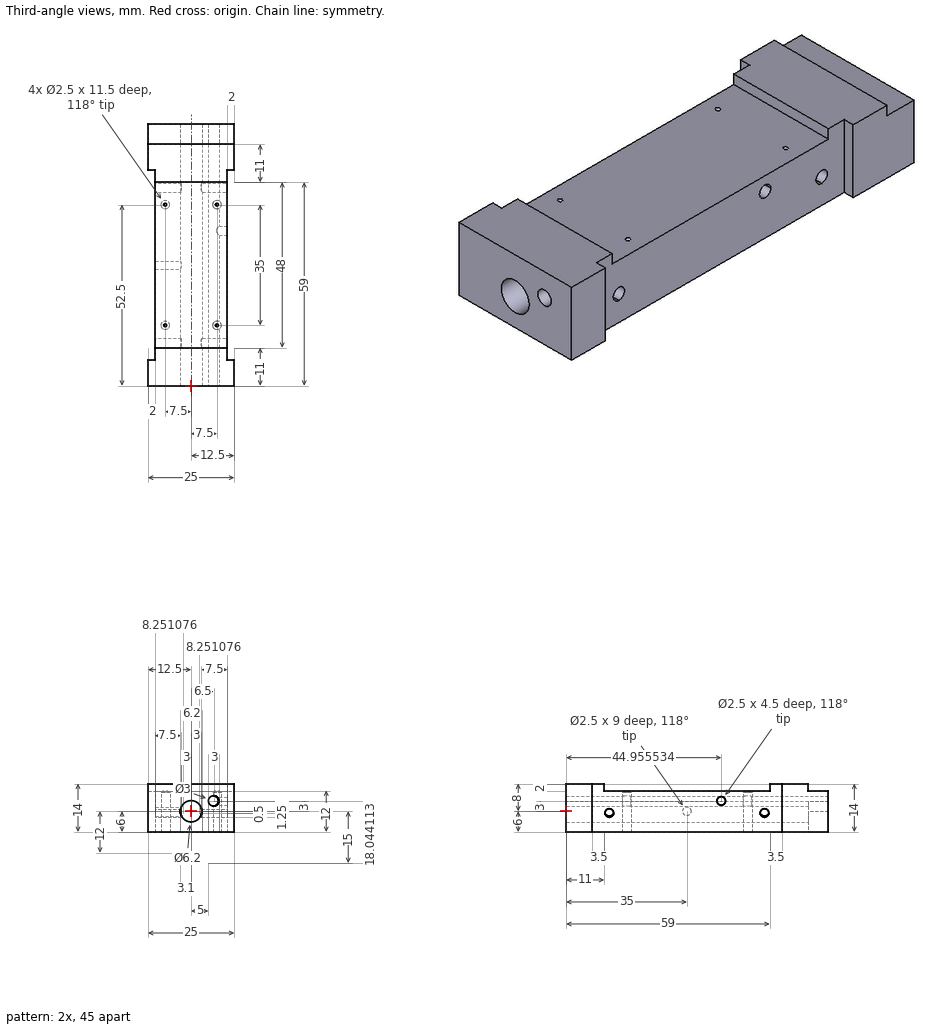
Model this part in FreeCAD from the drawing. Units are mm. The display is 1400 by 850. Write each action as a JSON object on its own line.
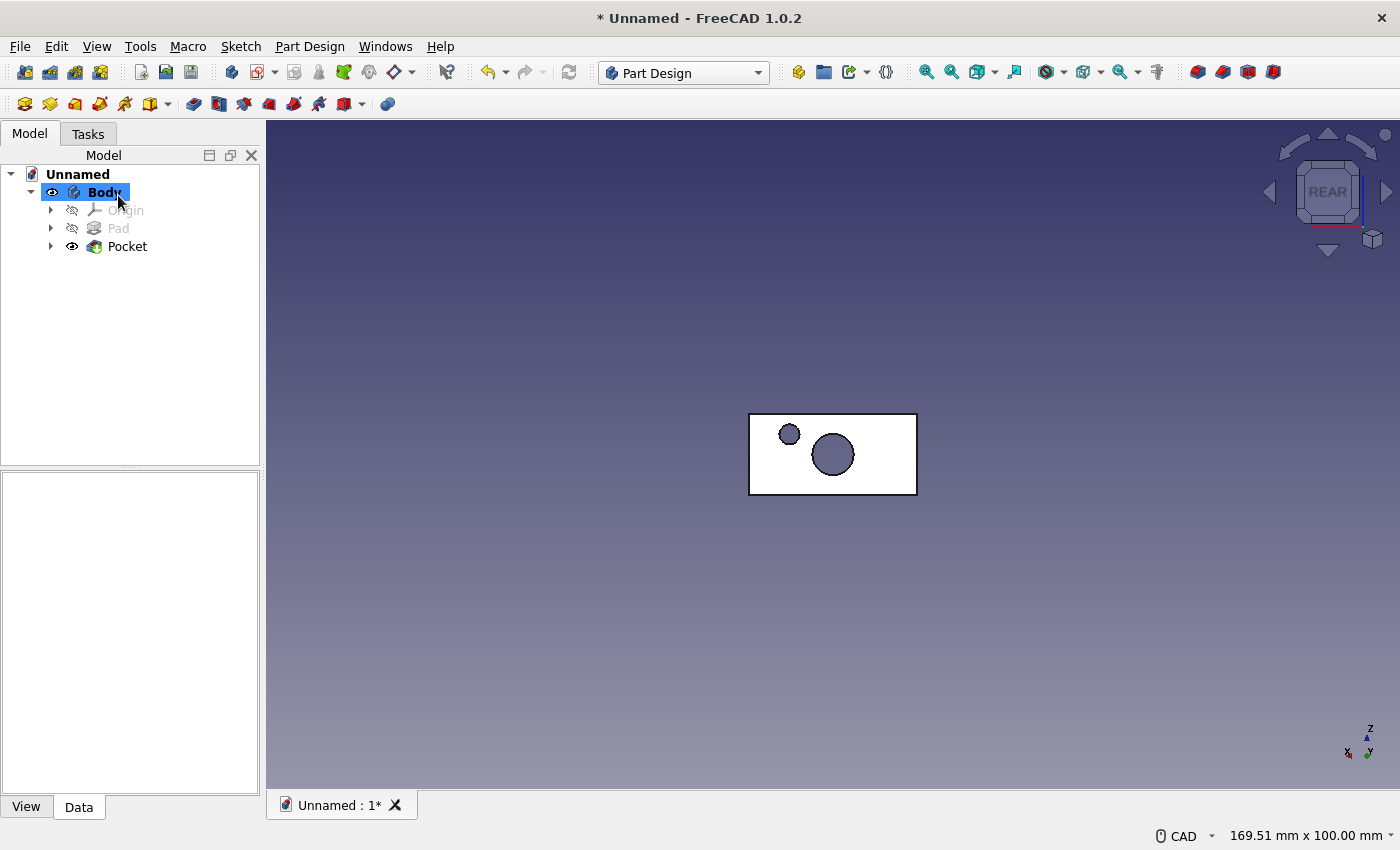
{"action": "left_click", "coordinate": [927, 72]}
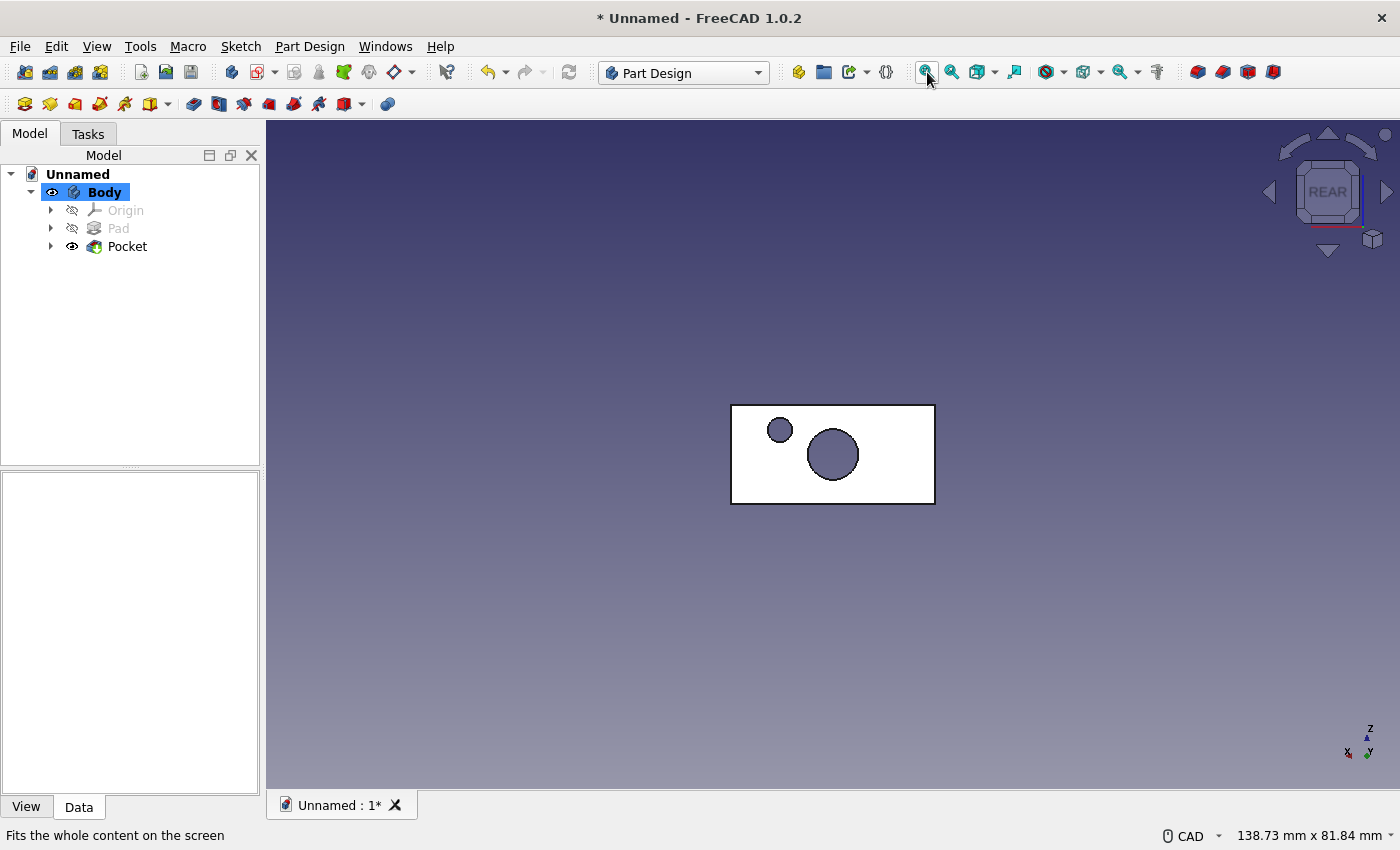
{"action": "left_click", "coordinate": [891, 439]}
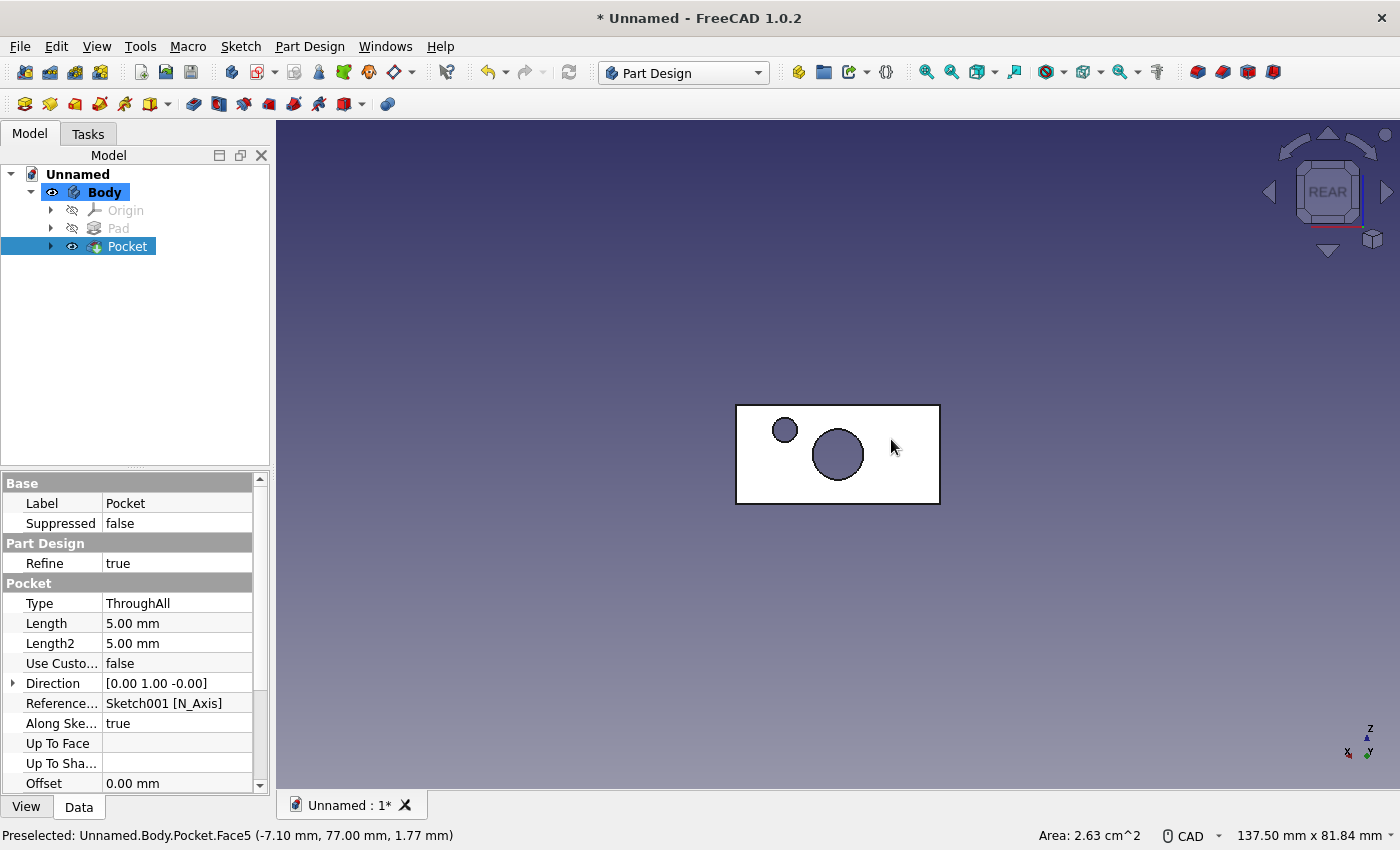
{"action": "left_click", "coordinate": [256, 72]}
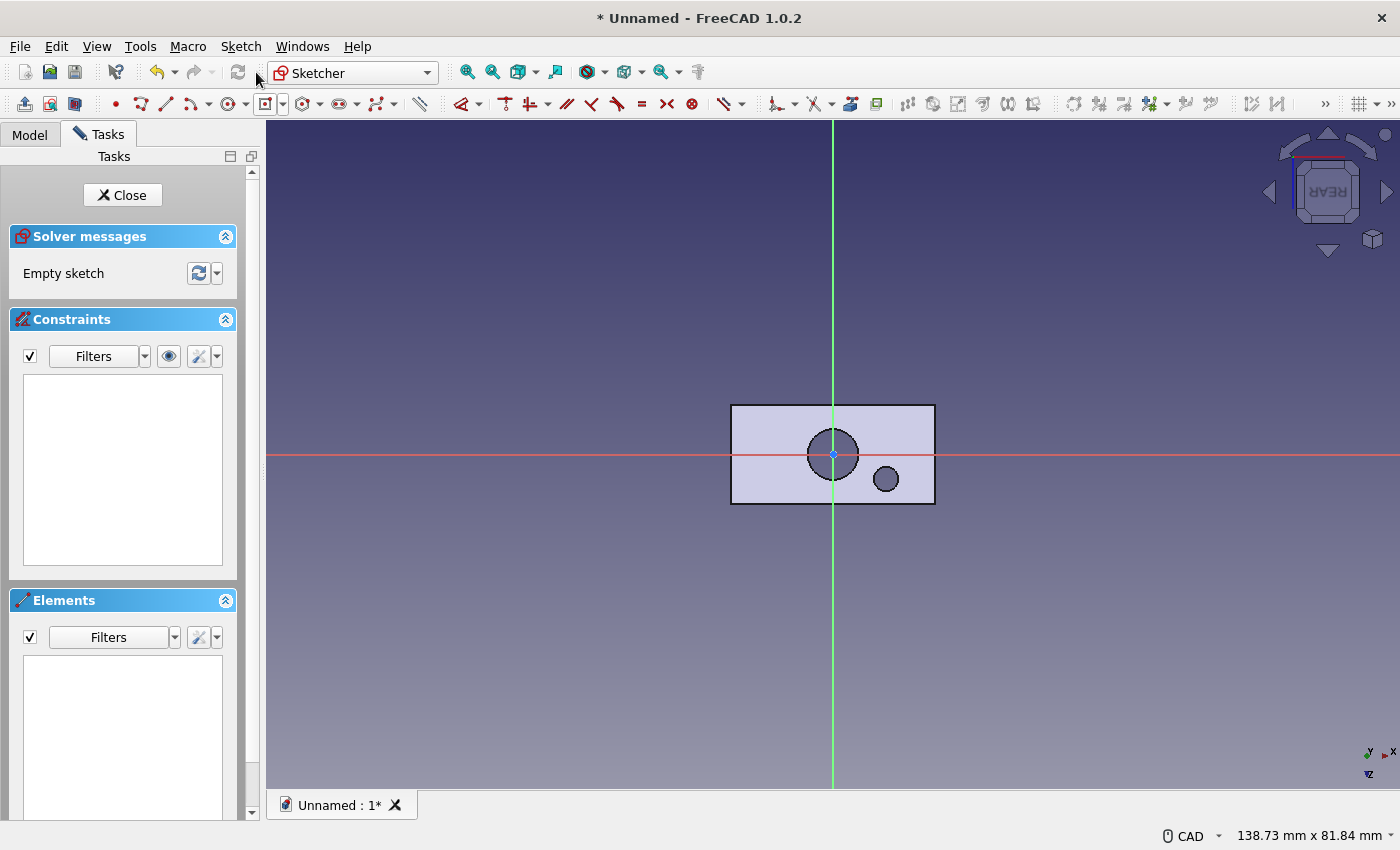
{"action": "scroll", "coordinate": [905, 377], "scroll_direction": "up", "scroll_amount": 5}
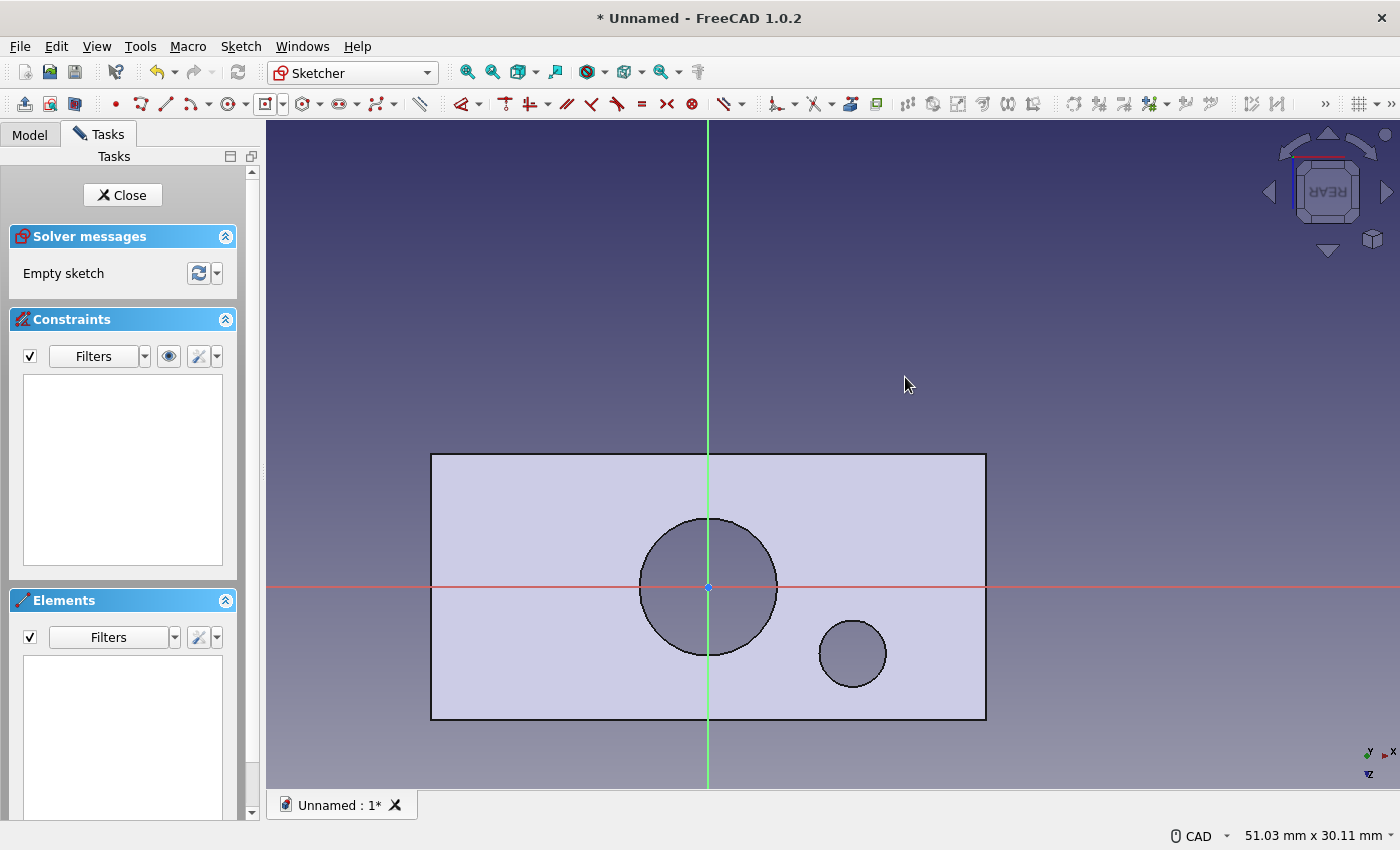
{"action": "left_click", "coordinate": [282, 104]}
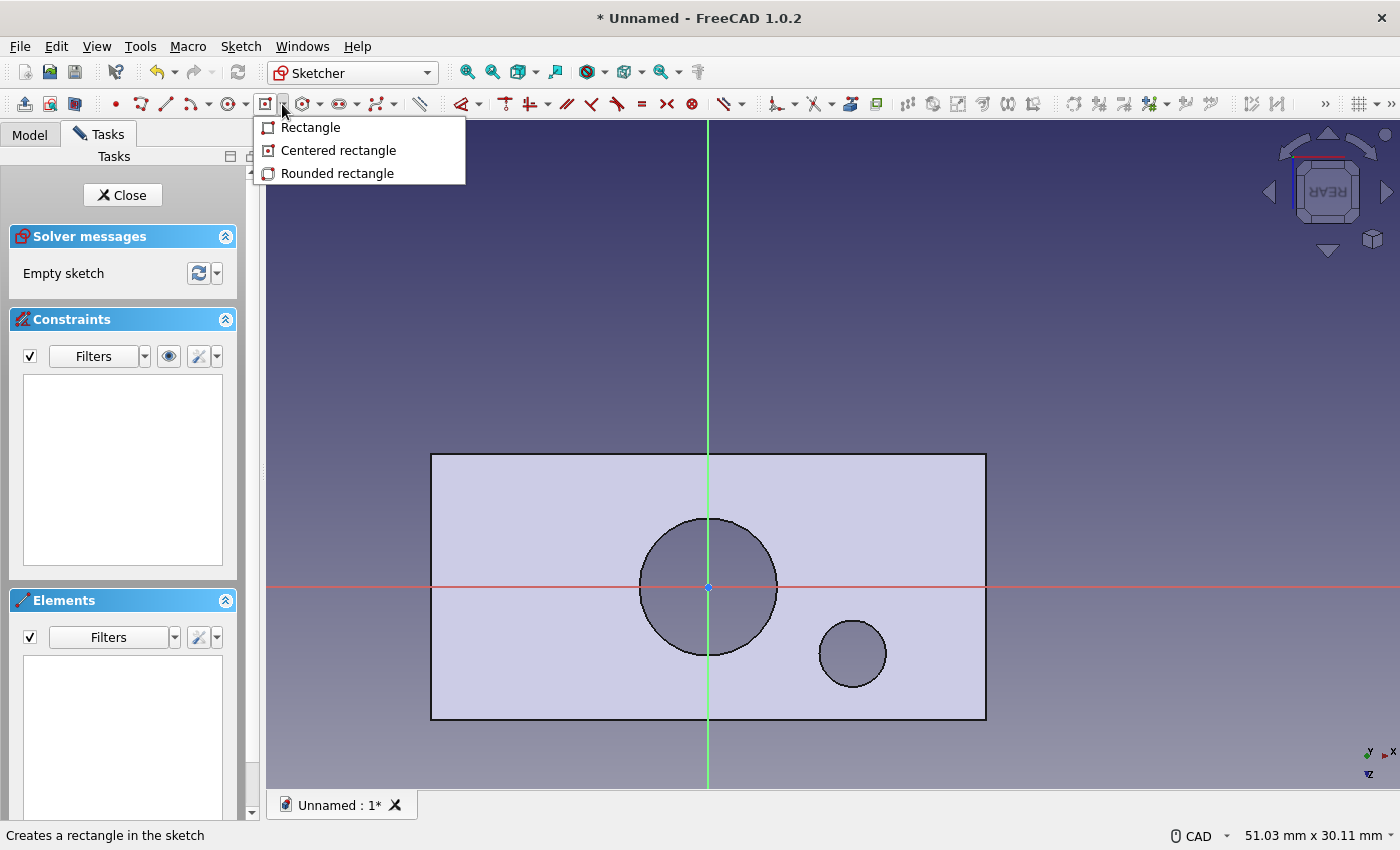
{"action": "left_click", "coordinate": [360, 128]}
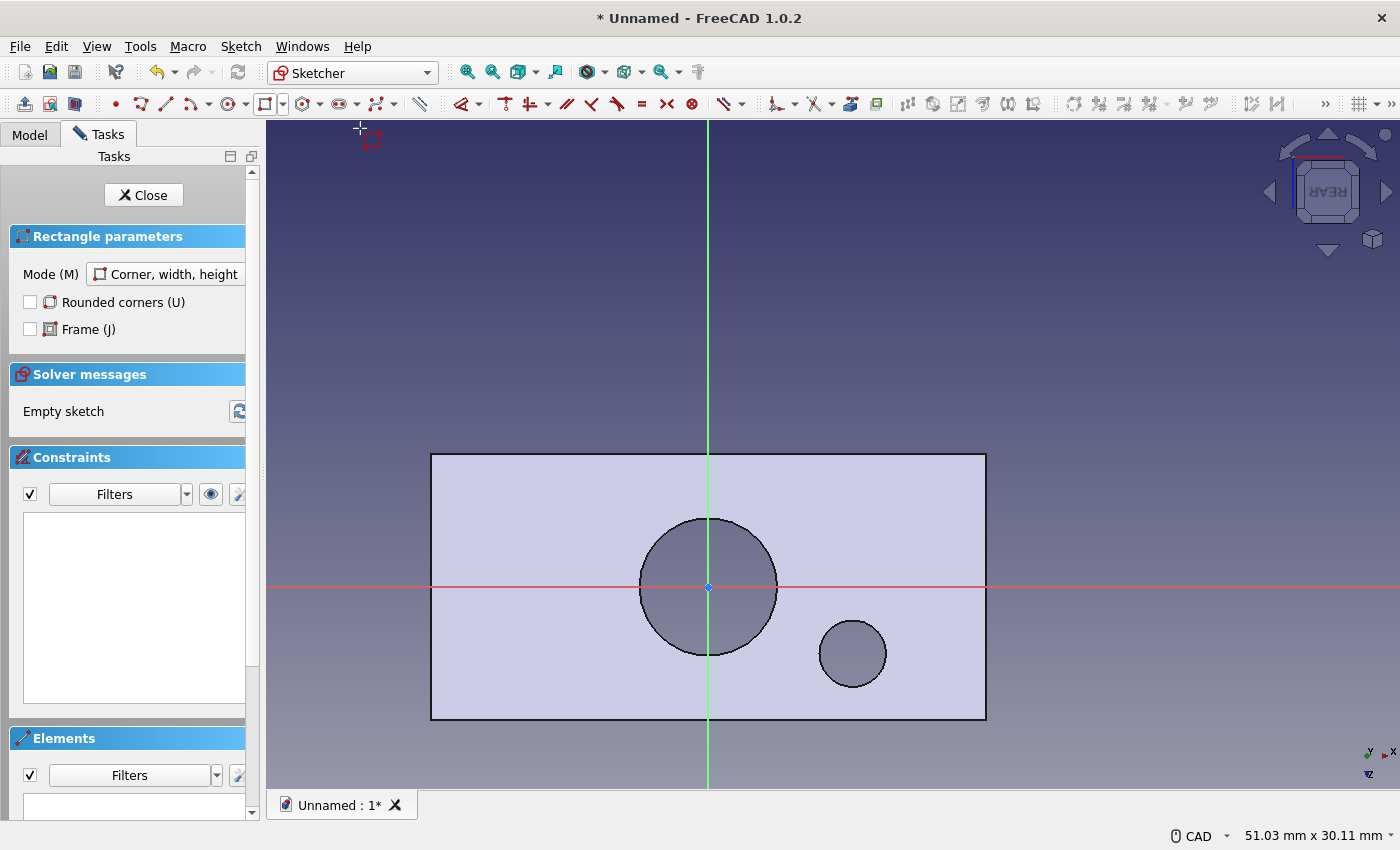
{"action": "left_click", "coordinate": [639, 320]}
{"action": "left_click", "coordinate": [777, 587]}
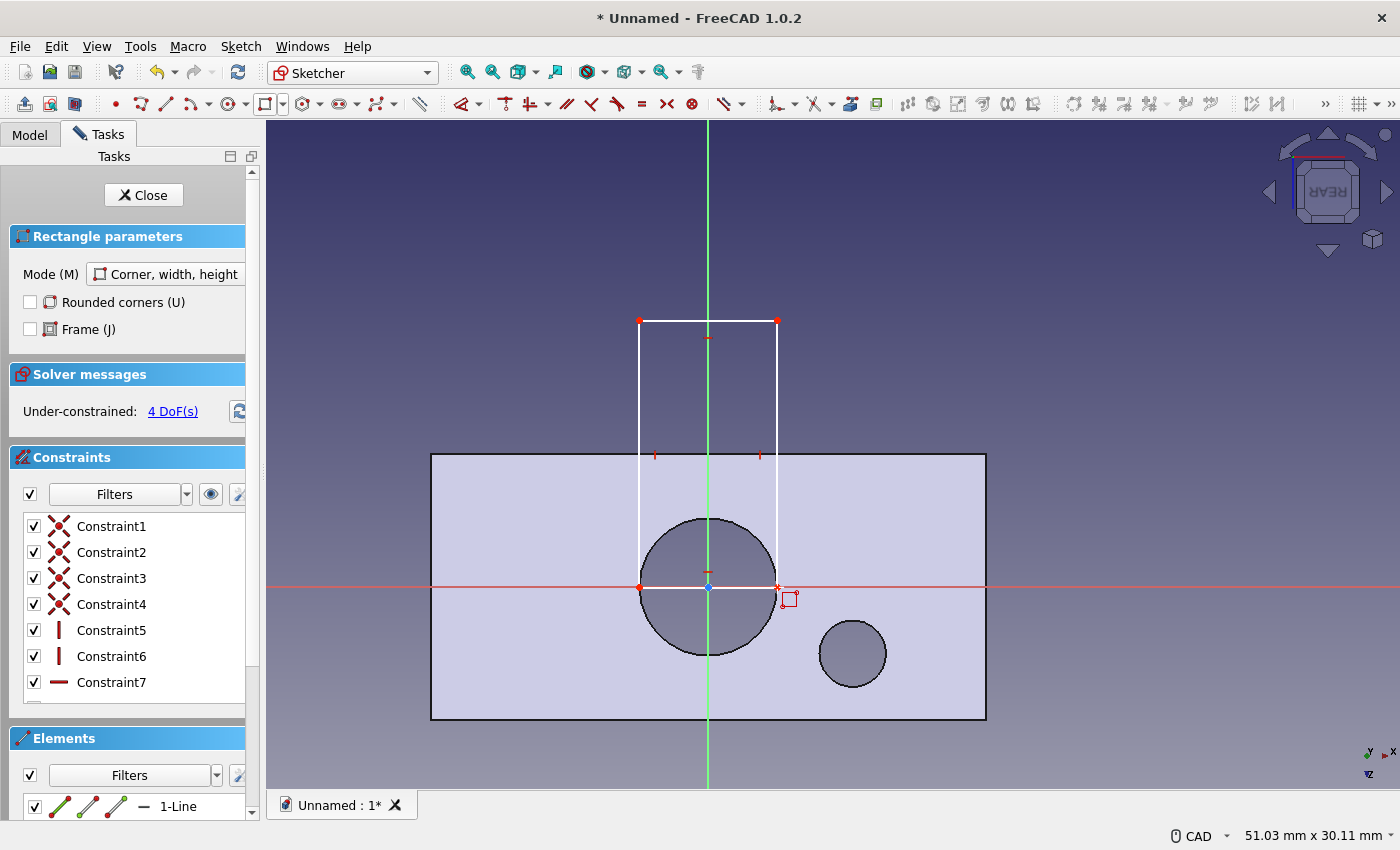
{"action": "left_click", "coordinate": [819, 254]}
{"action": "left_click", "coordinate": [886, 655]}
{"action": "key", "text": "Escape"}